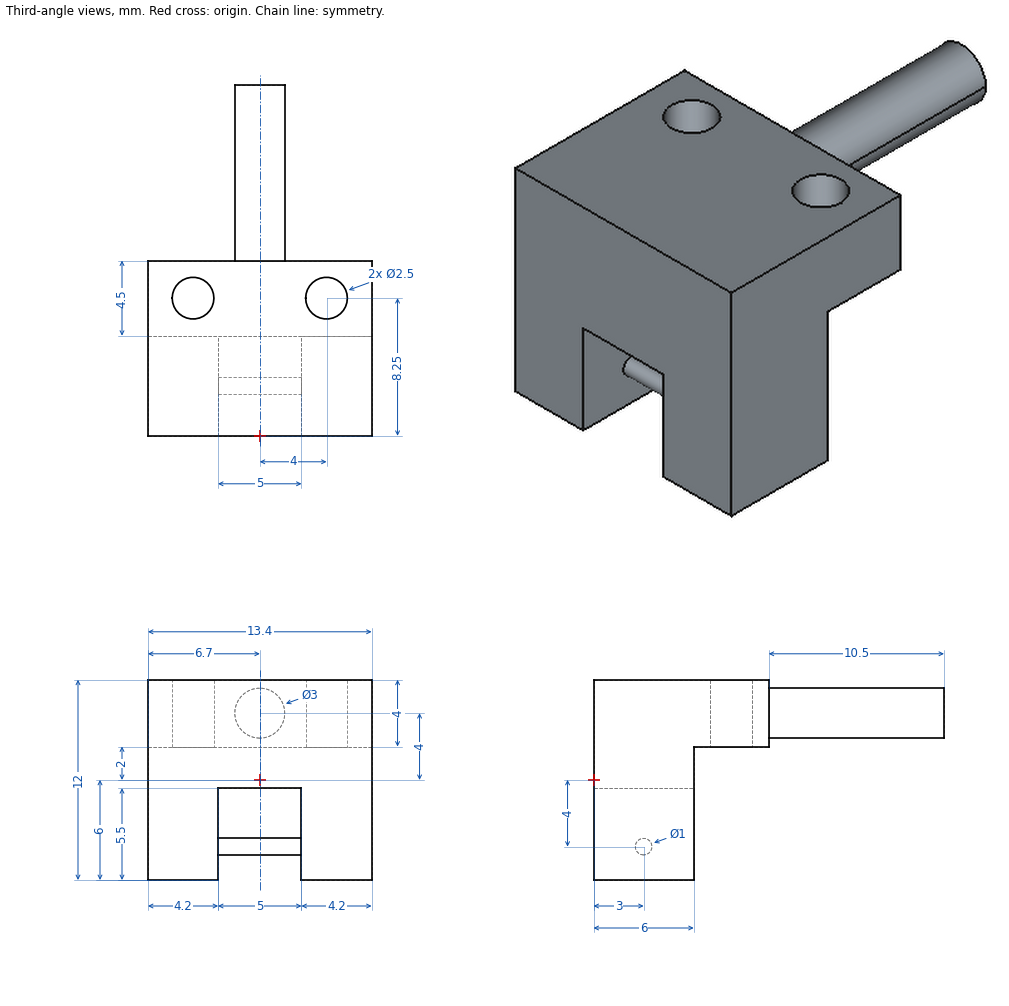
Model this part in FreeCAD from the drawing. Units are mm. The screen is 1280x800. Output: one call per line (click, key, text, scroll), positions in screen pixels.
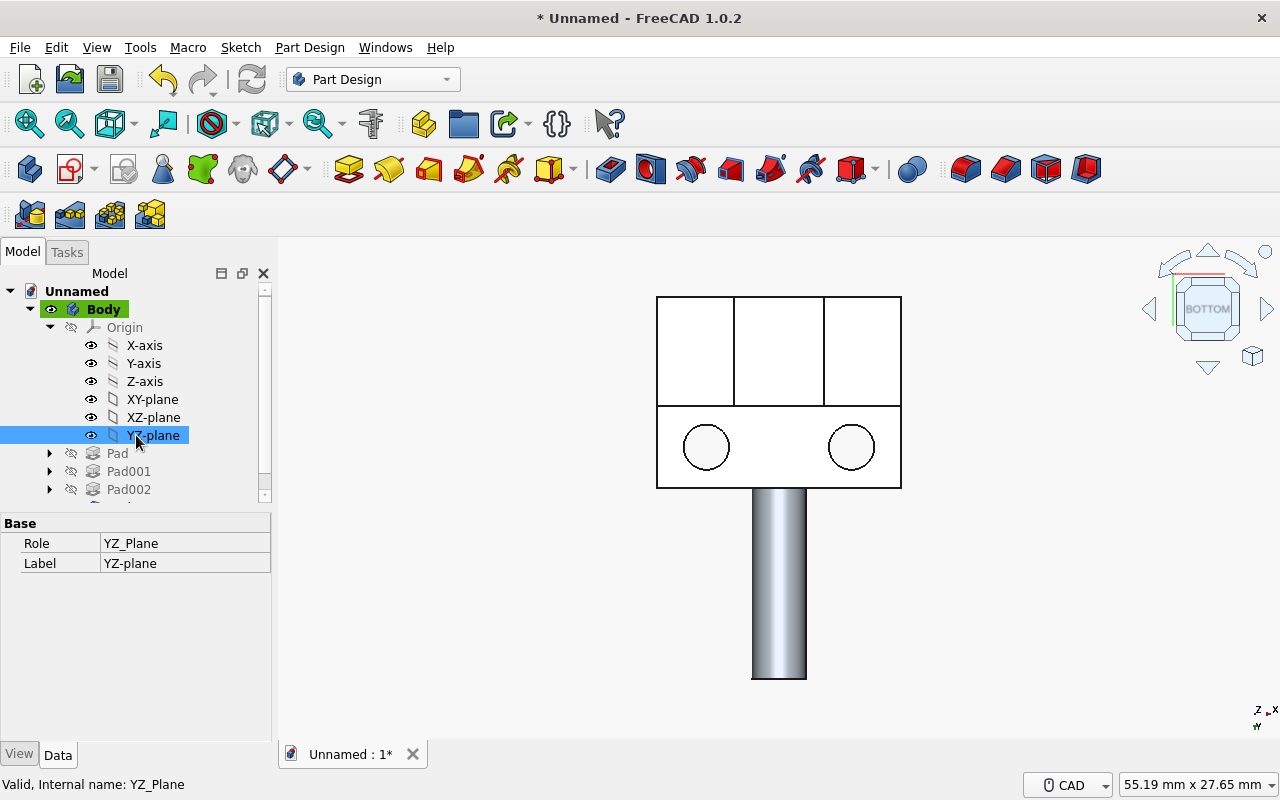
click(284, 170)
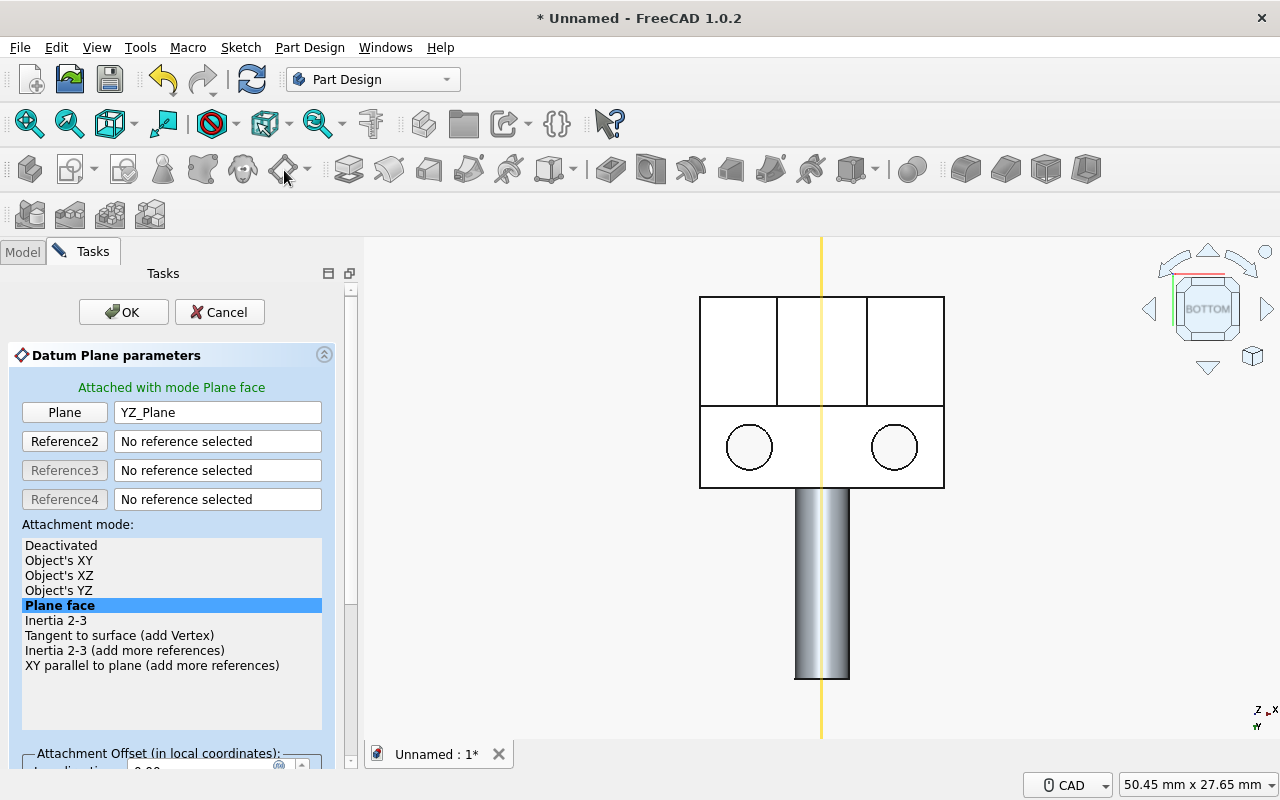
scroll(351, 526, down, 3)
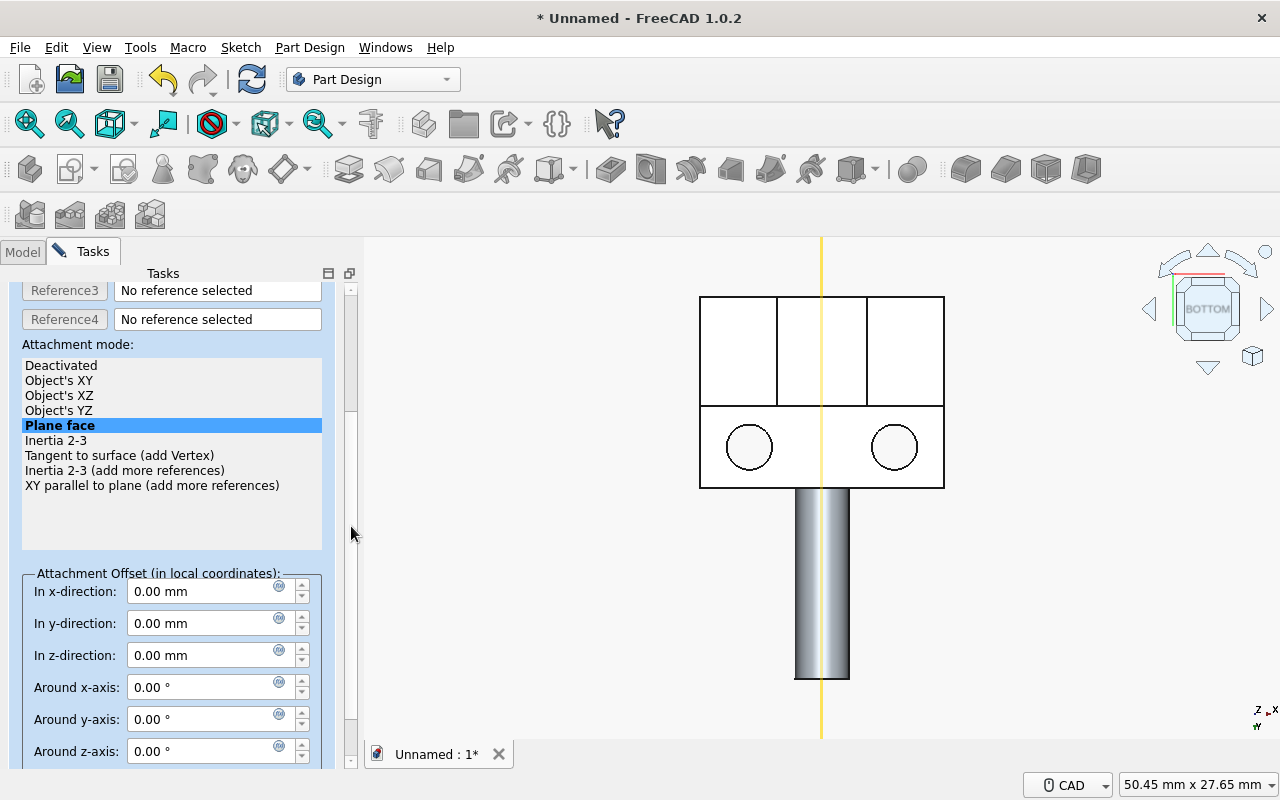
triple_click(210, 655)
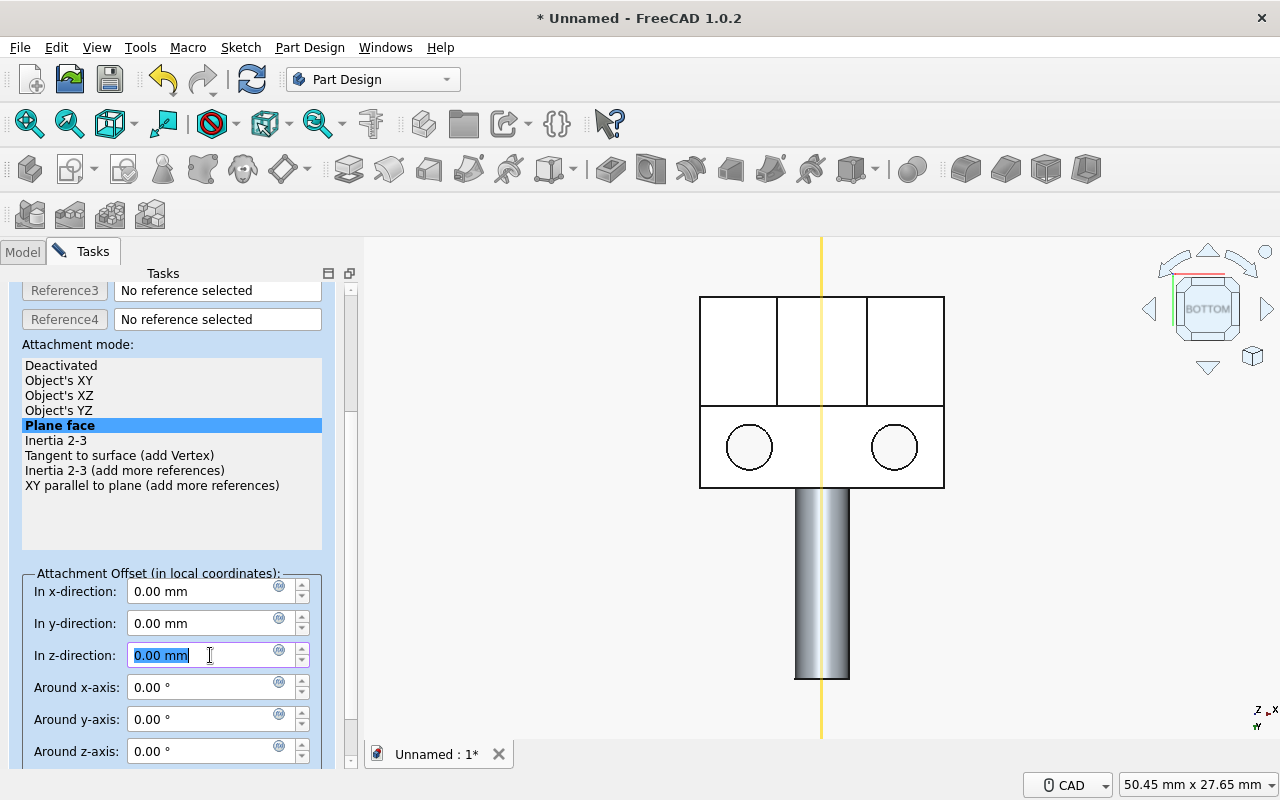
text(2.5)
key(Tab)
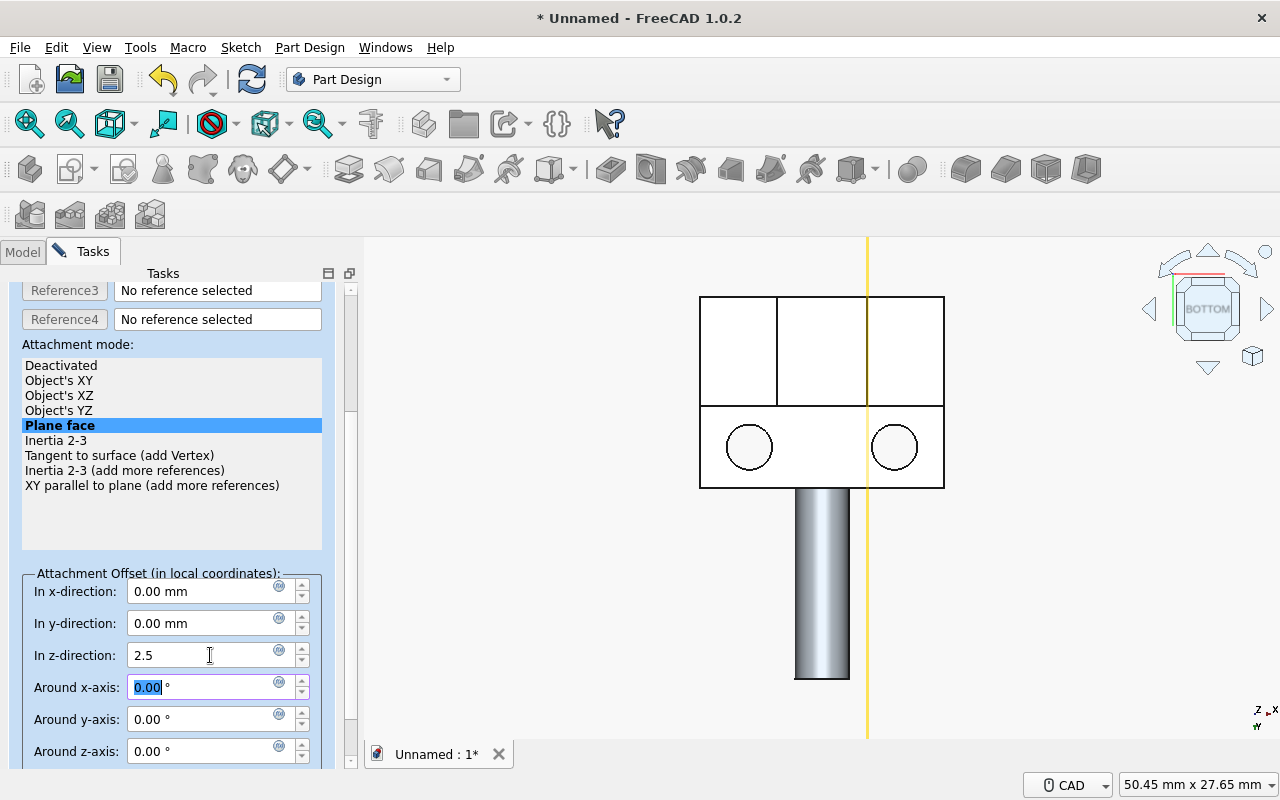
scroll(351, 526, up, 4)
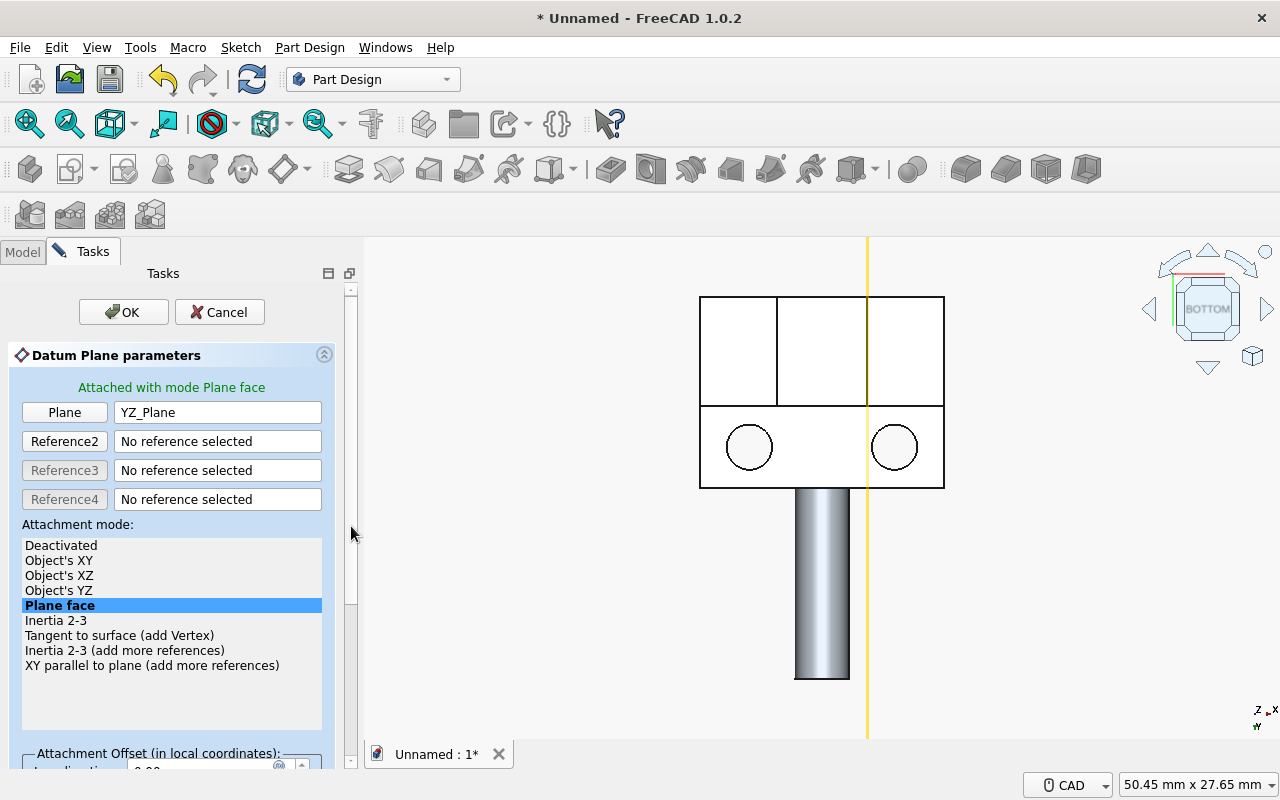
click(124, 312)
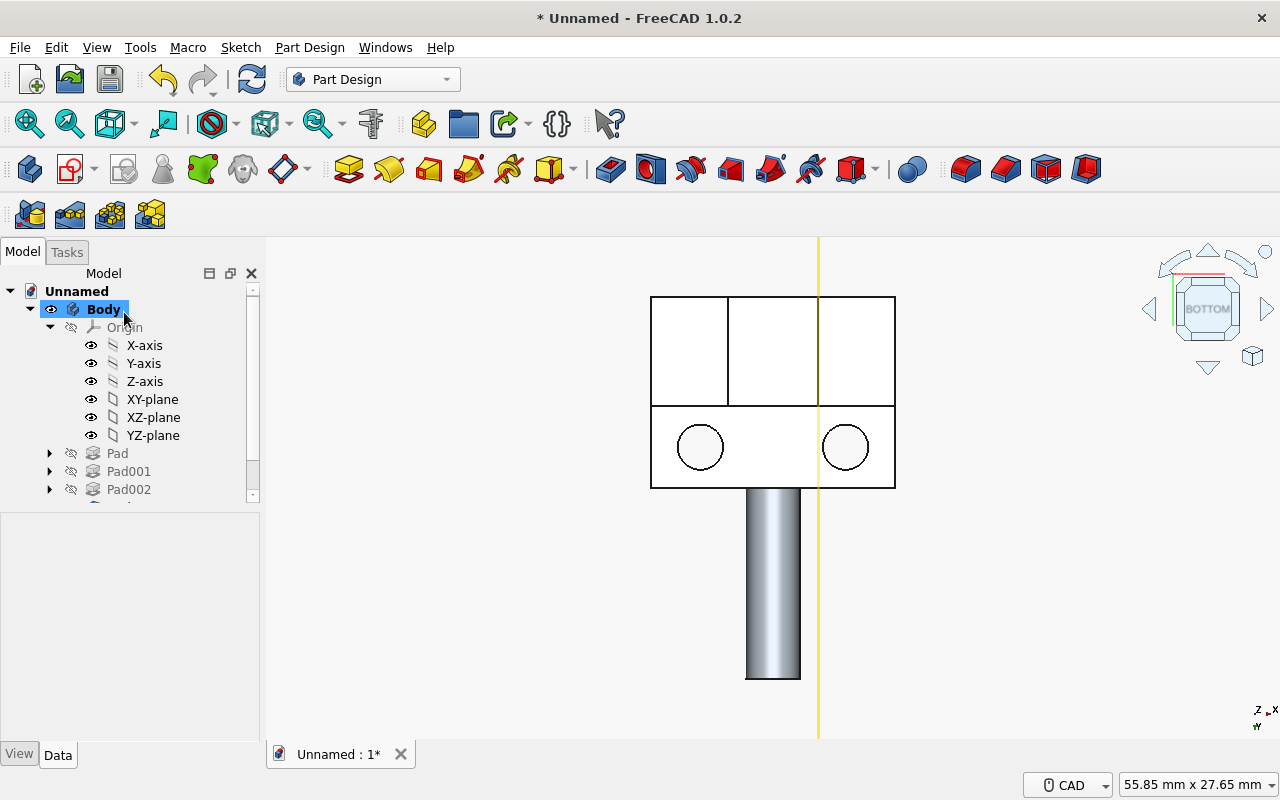
scroll(100, 395, down, 3)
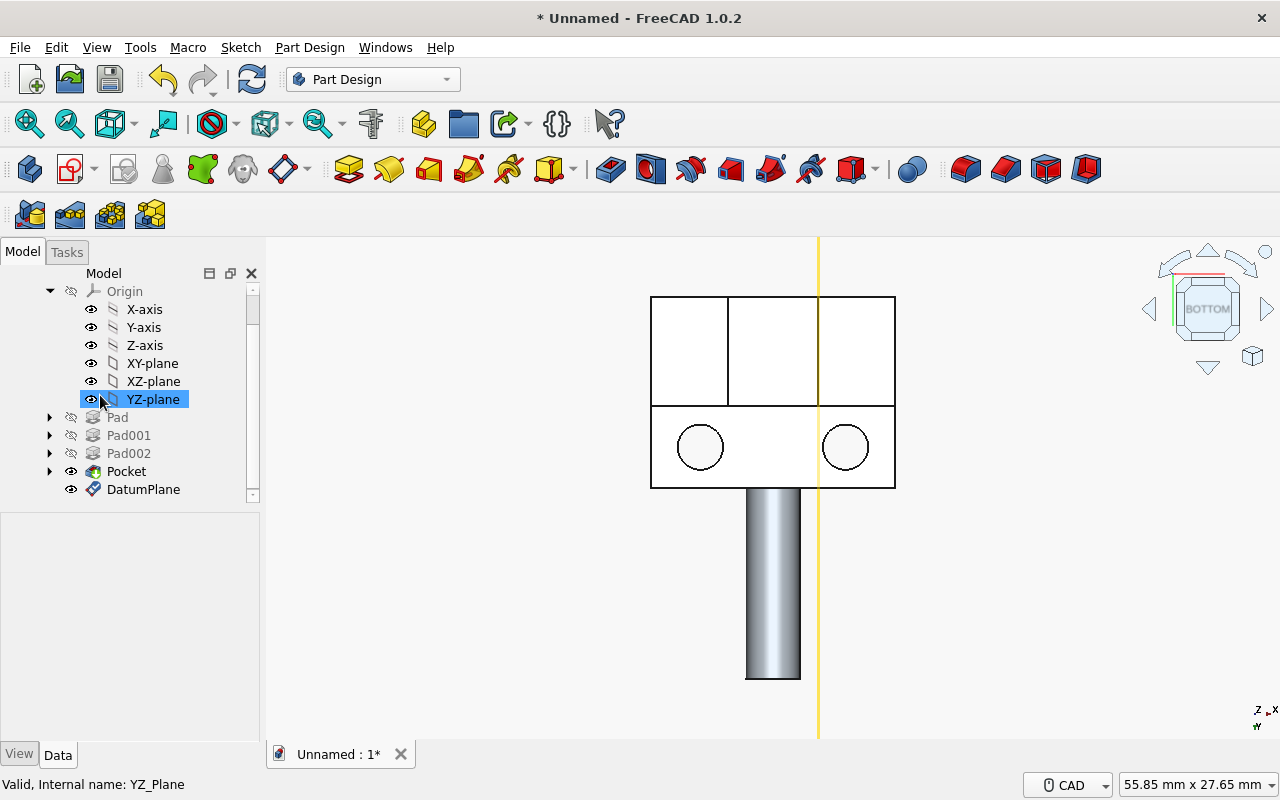
click(116, 489)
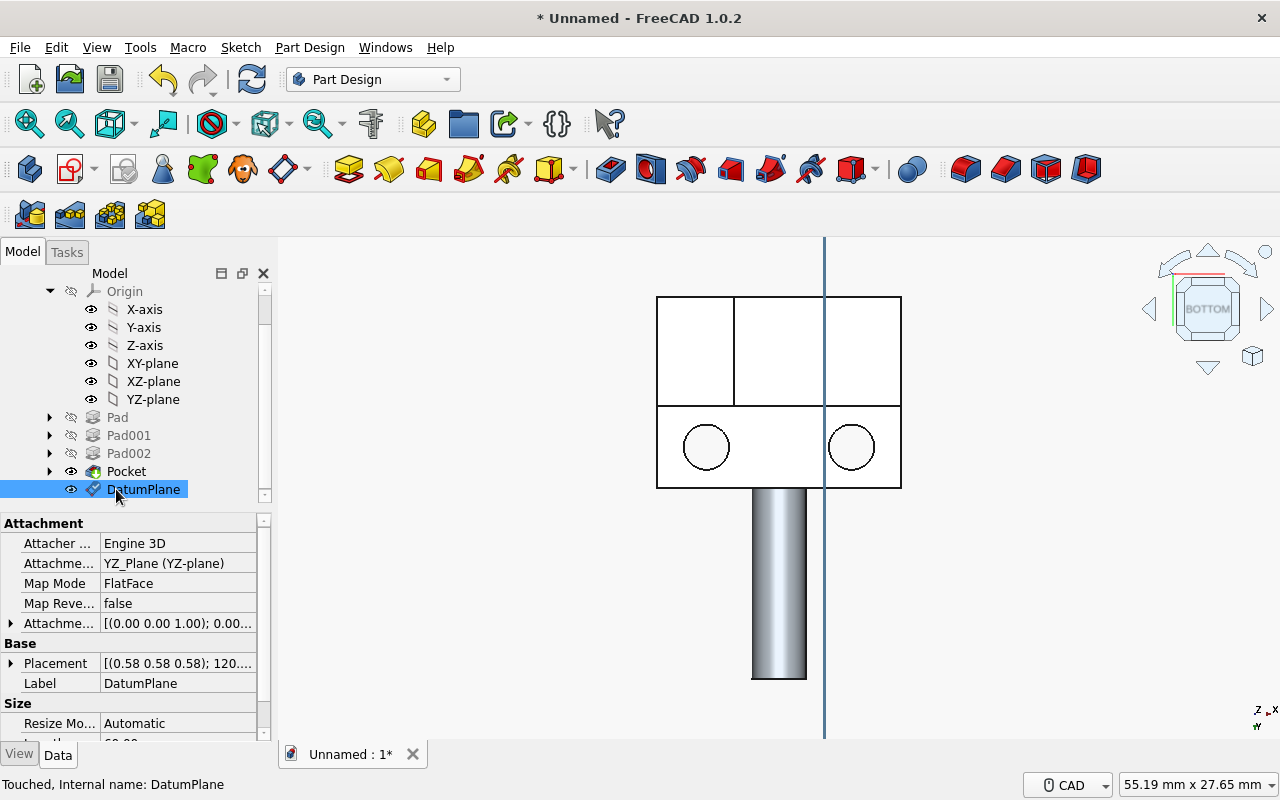
click(70, 170)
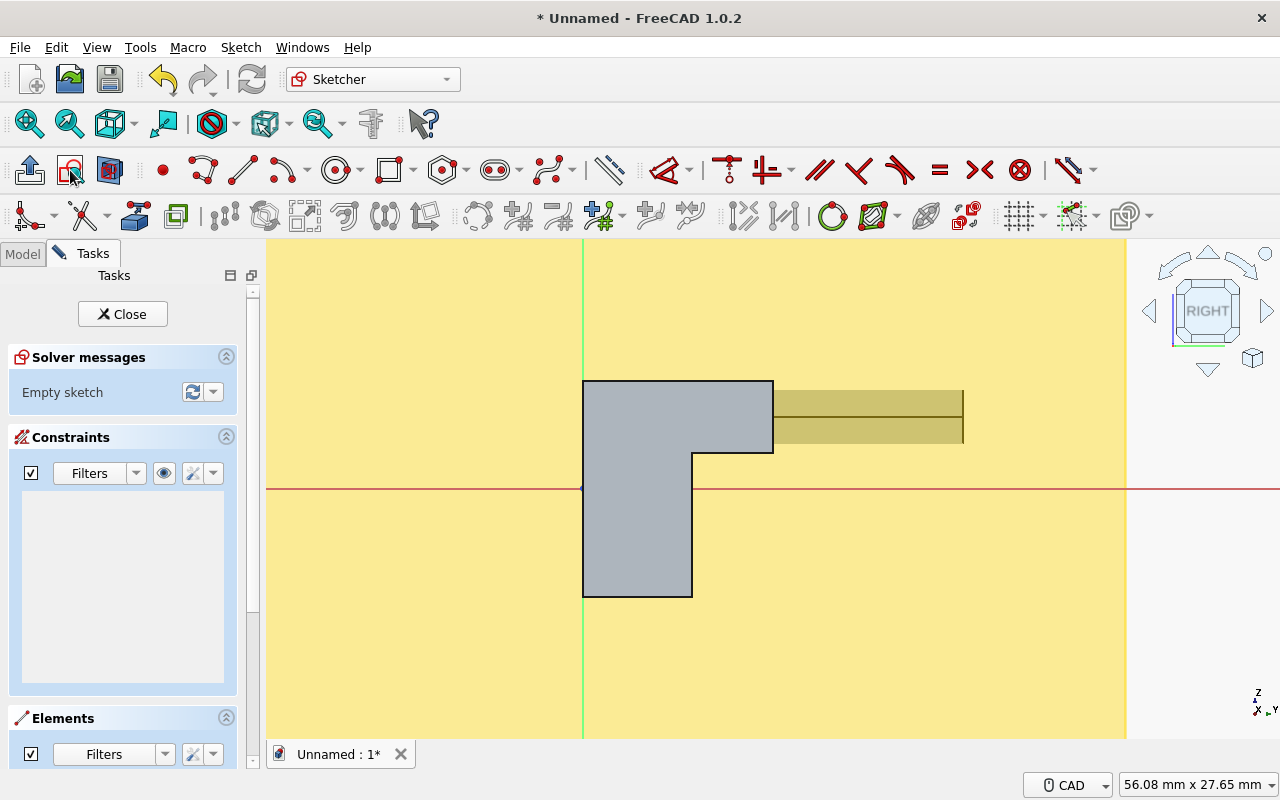
click(110, 170)